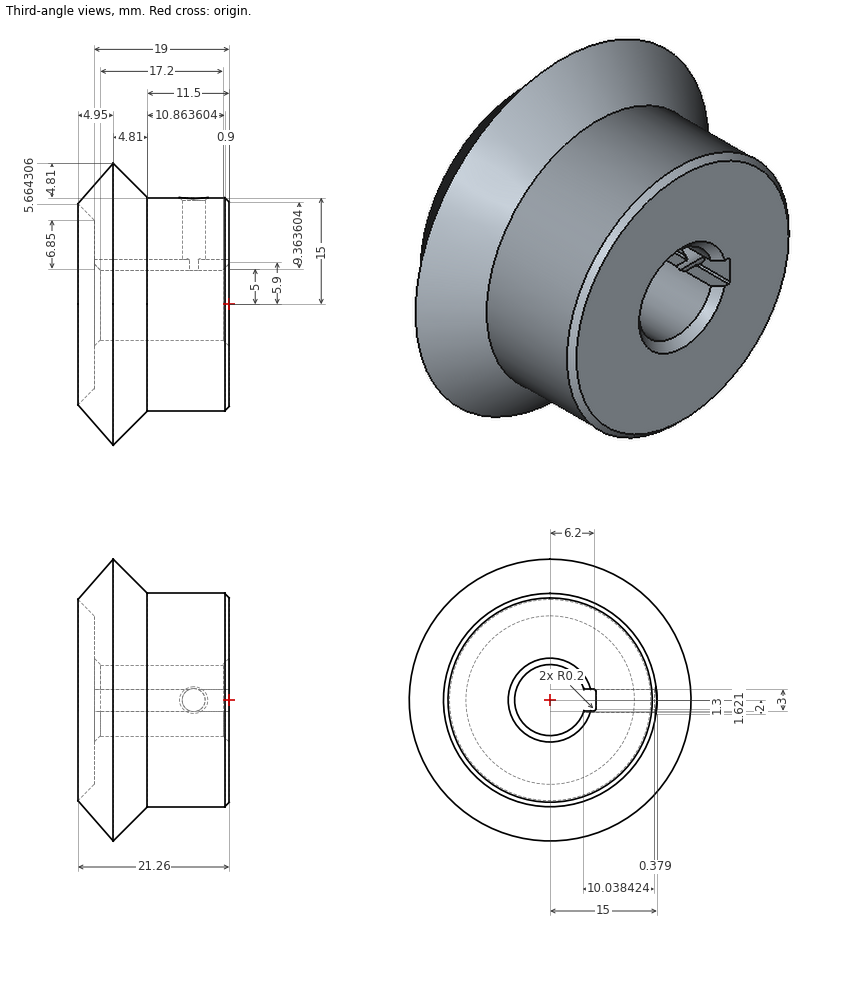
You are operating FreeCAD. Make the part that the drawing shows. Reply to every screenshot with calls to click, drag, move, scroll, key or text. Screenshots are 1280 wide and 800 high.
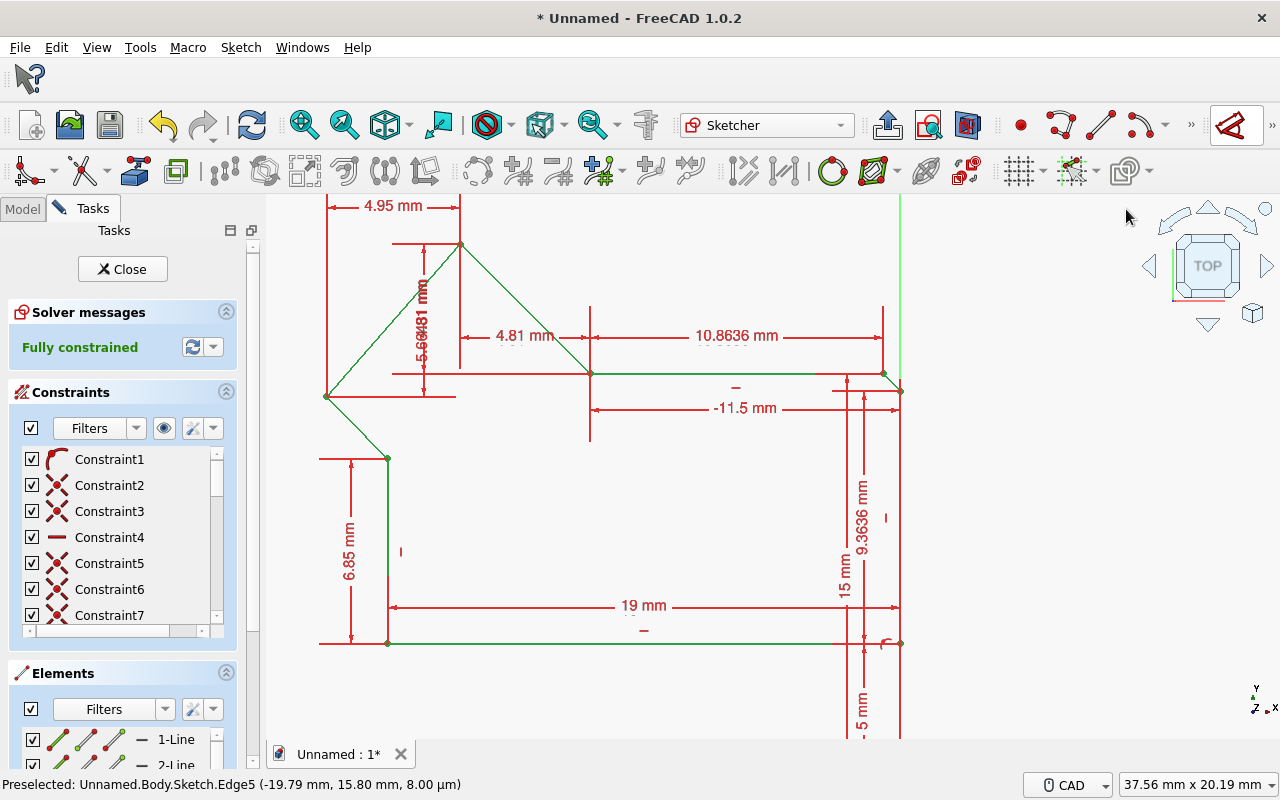
click(123, 269)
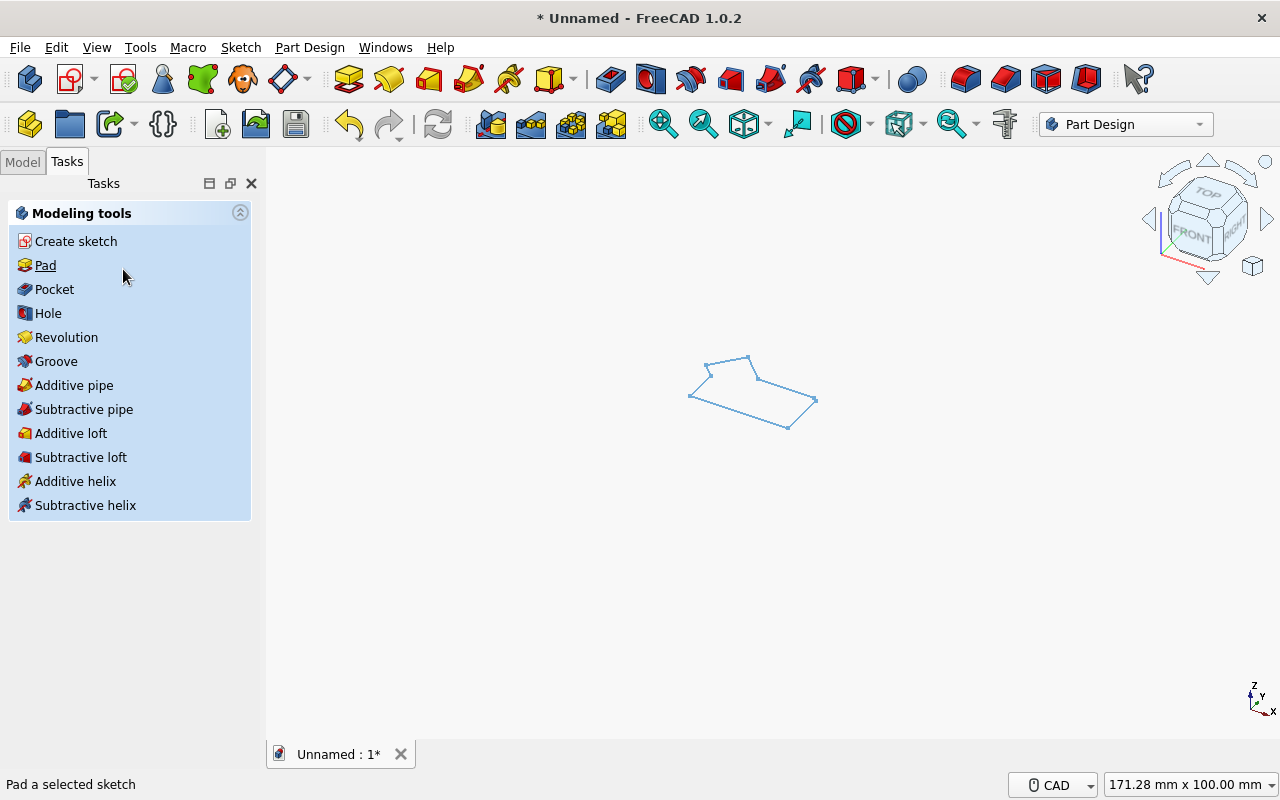
click(390, 80)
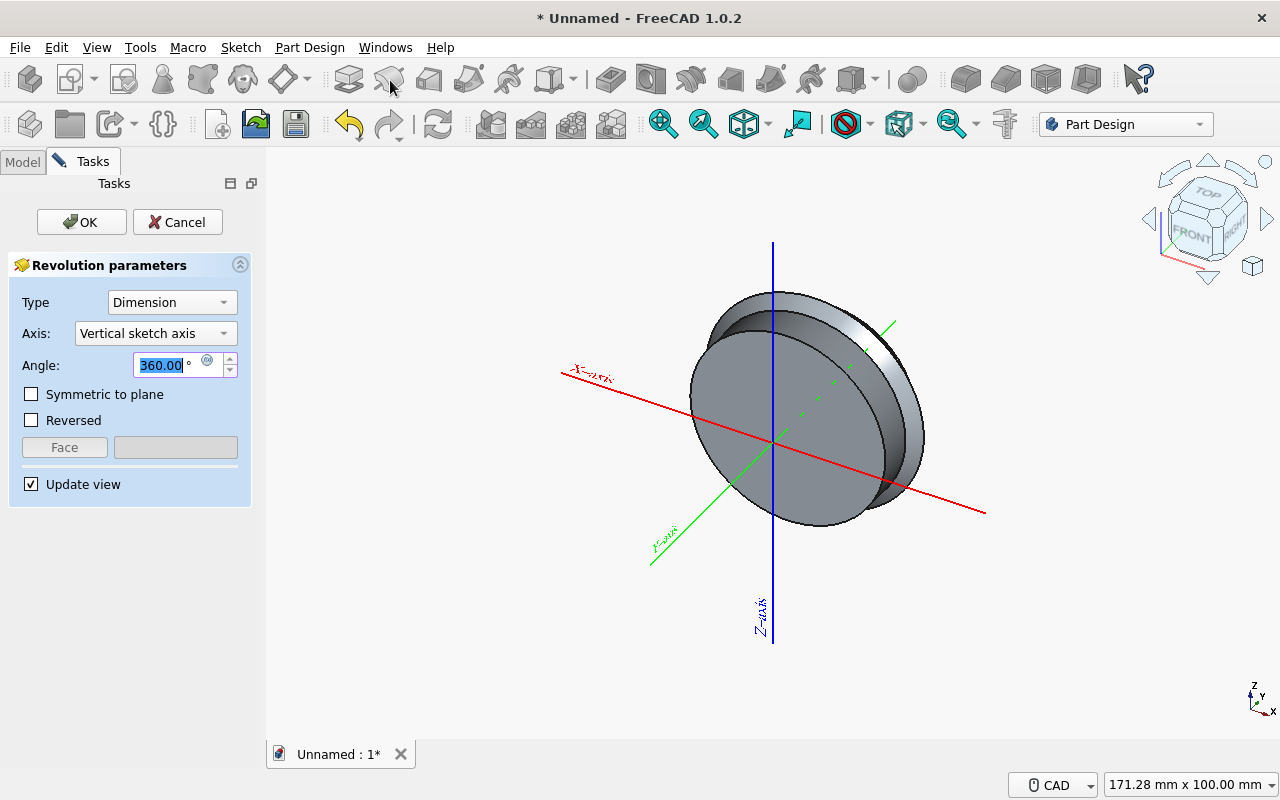
click(156, 334)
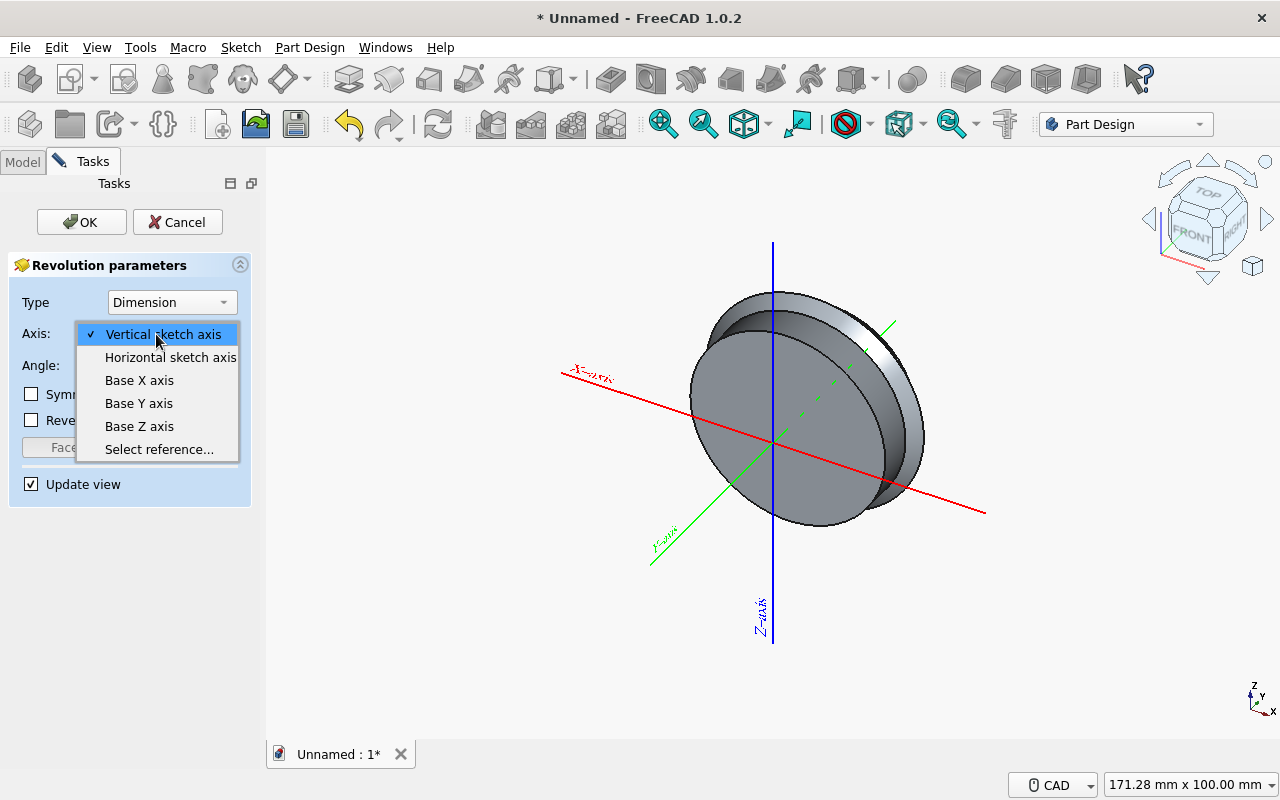
click(156, 358)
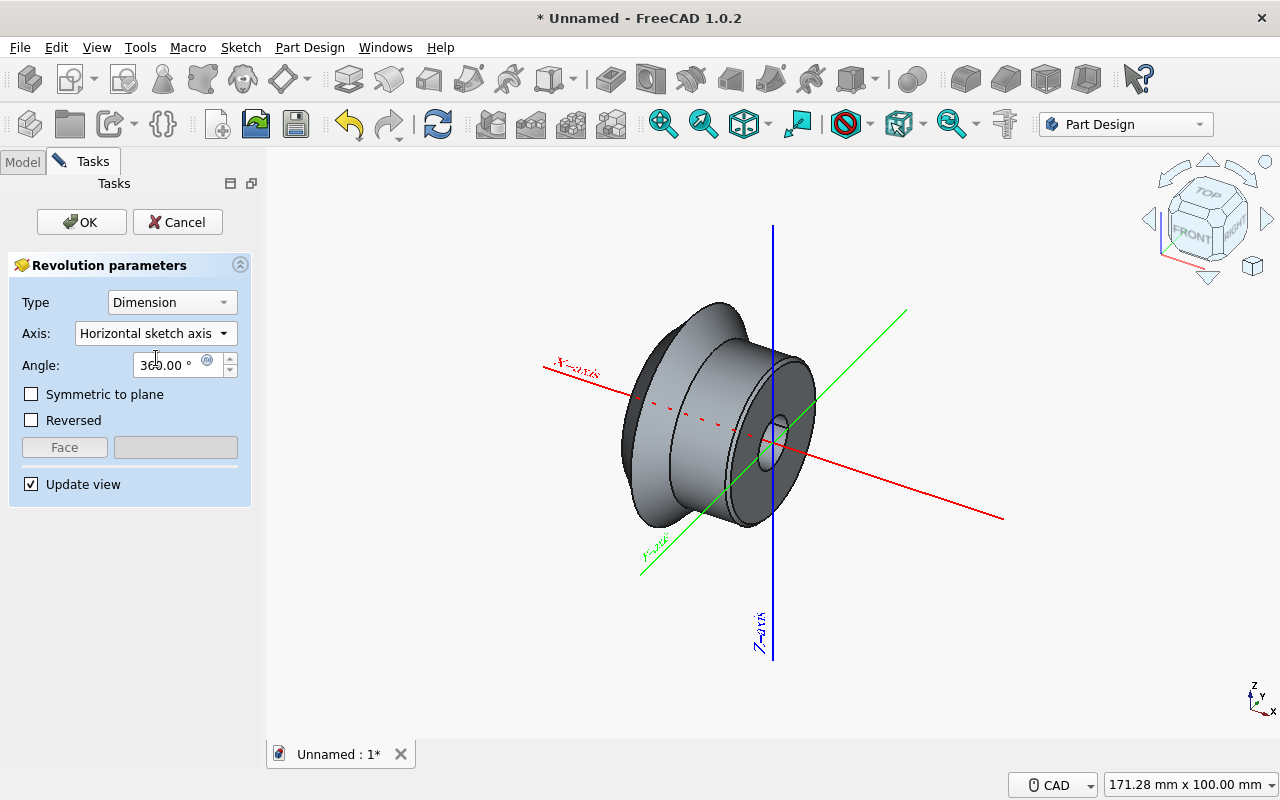
click(82, 222)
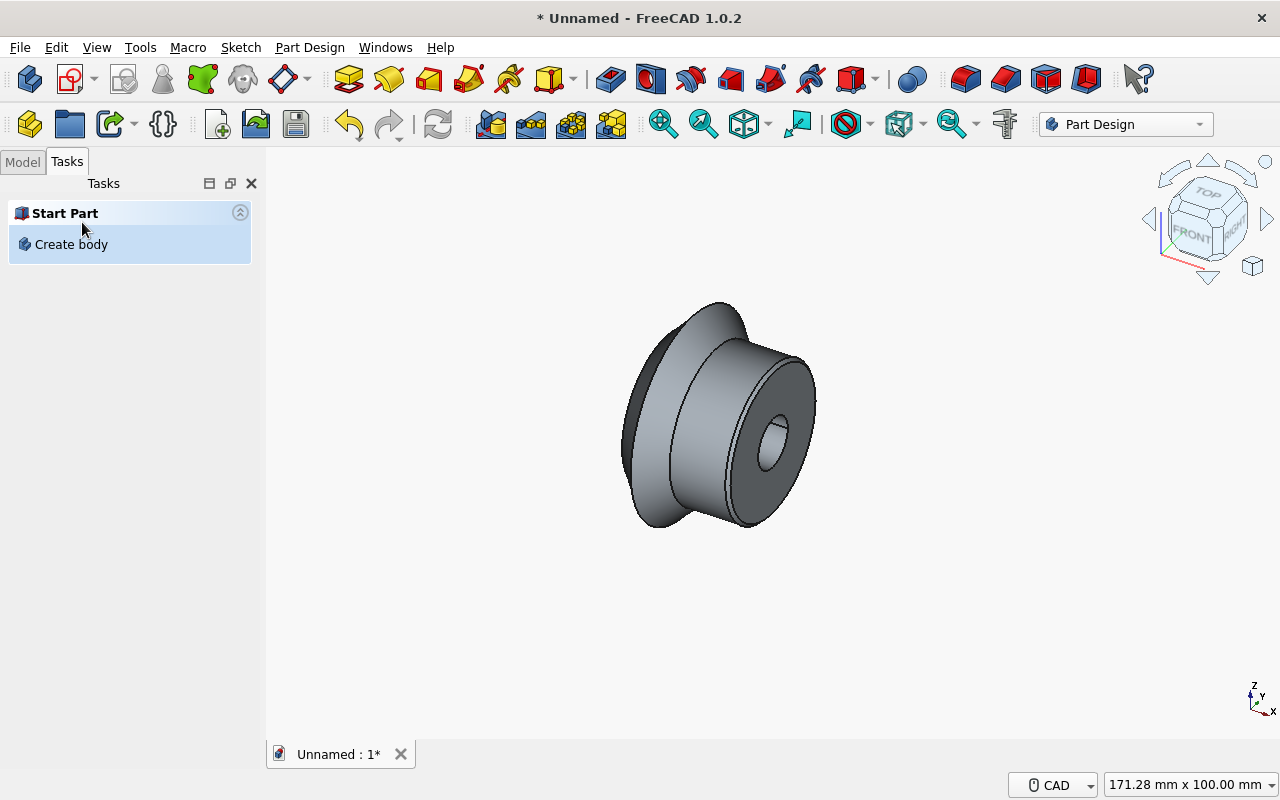
click(70, 80)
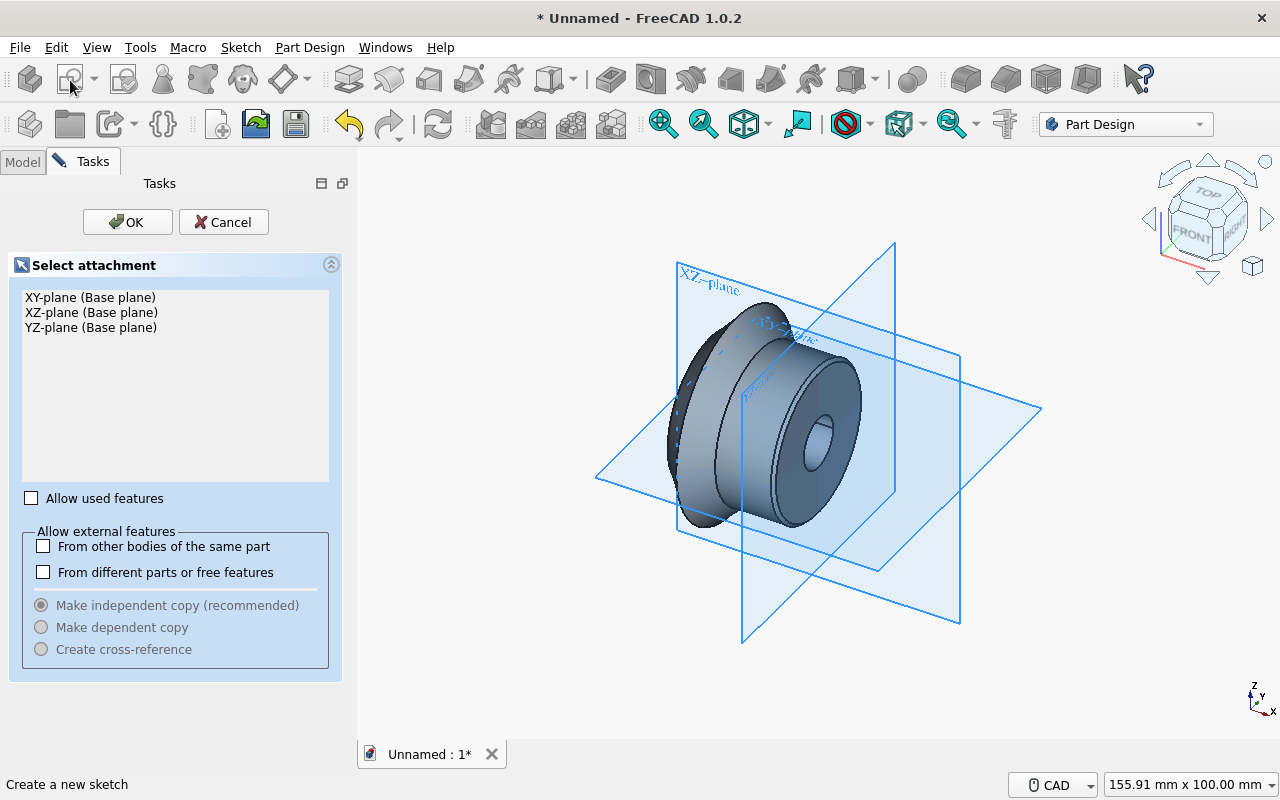
click(82, 298)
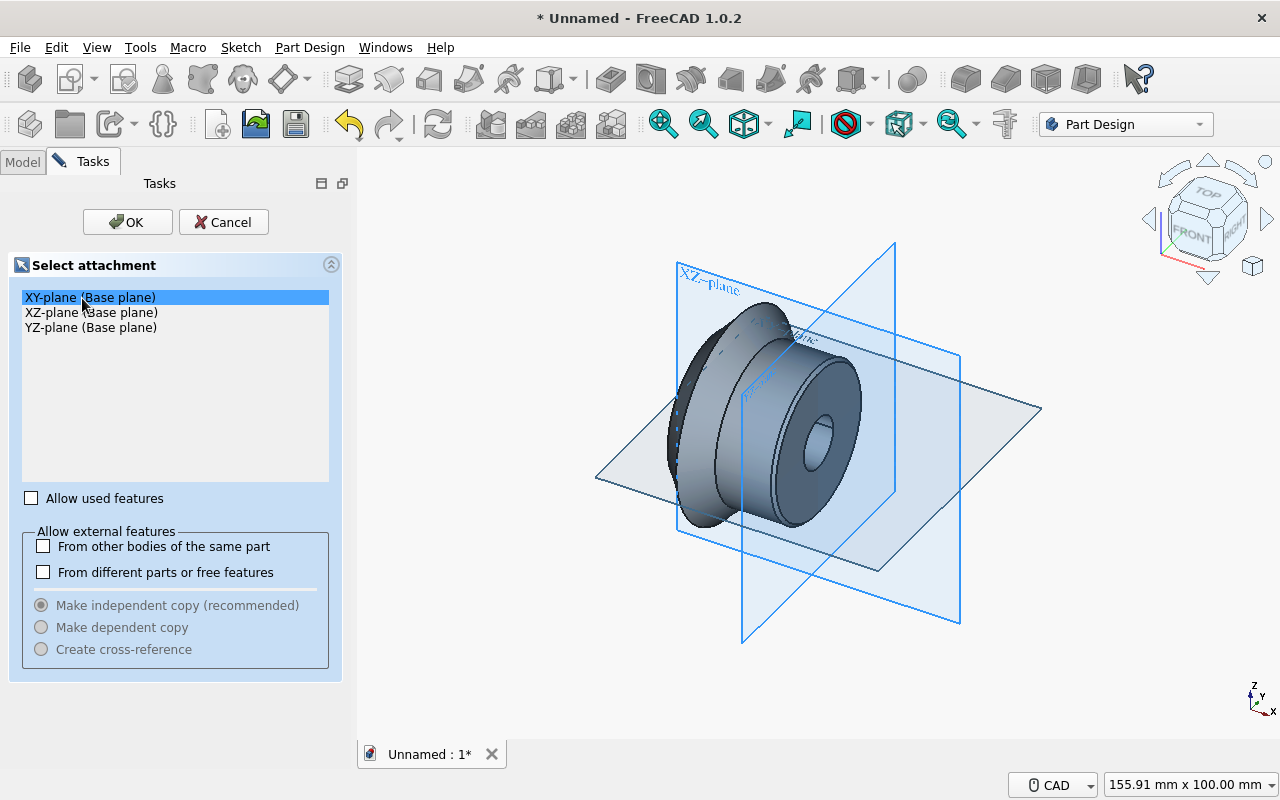
click(128, 222)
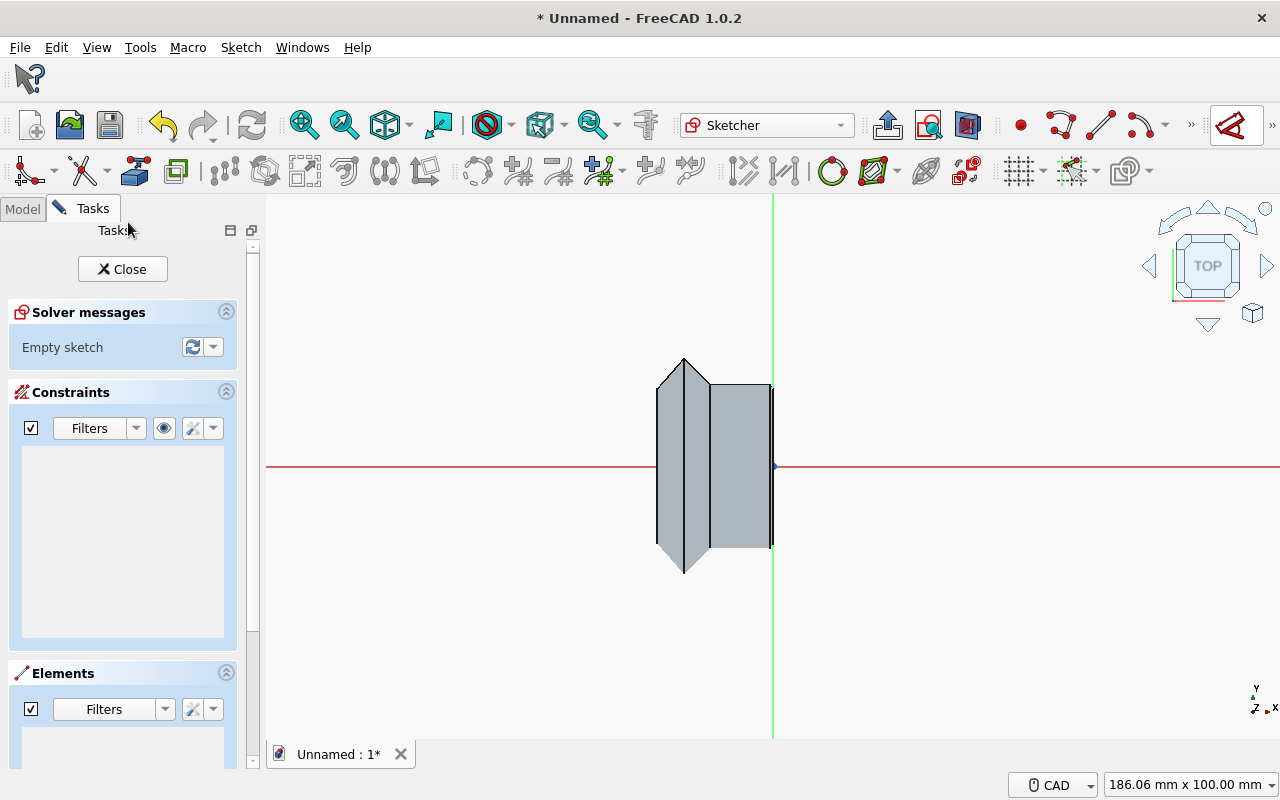
click(968, 126)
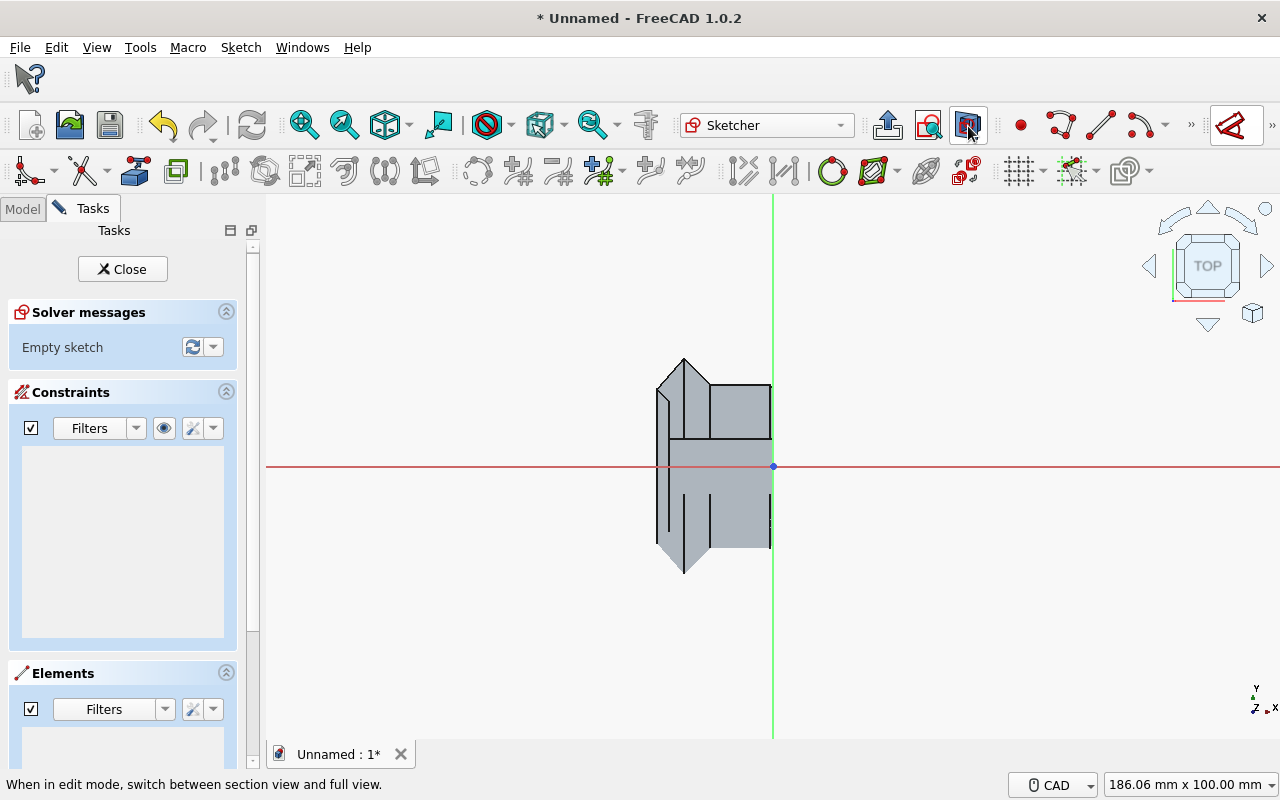
scroll(725, 447, up, 9)